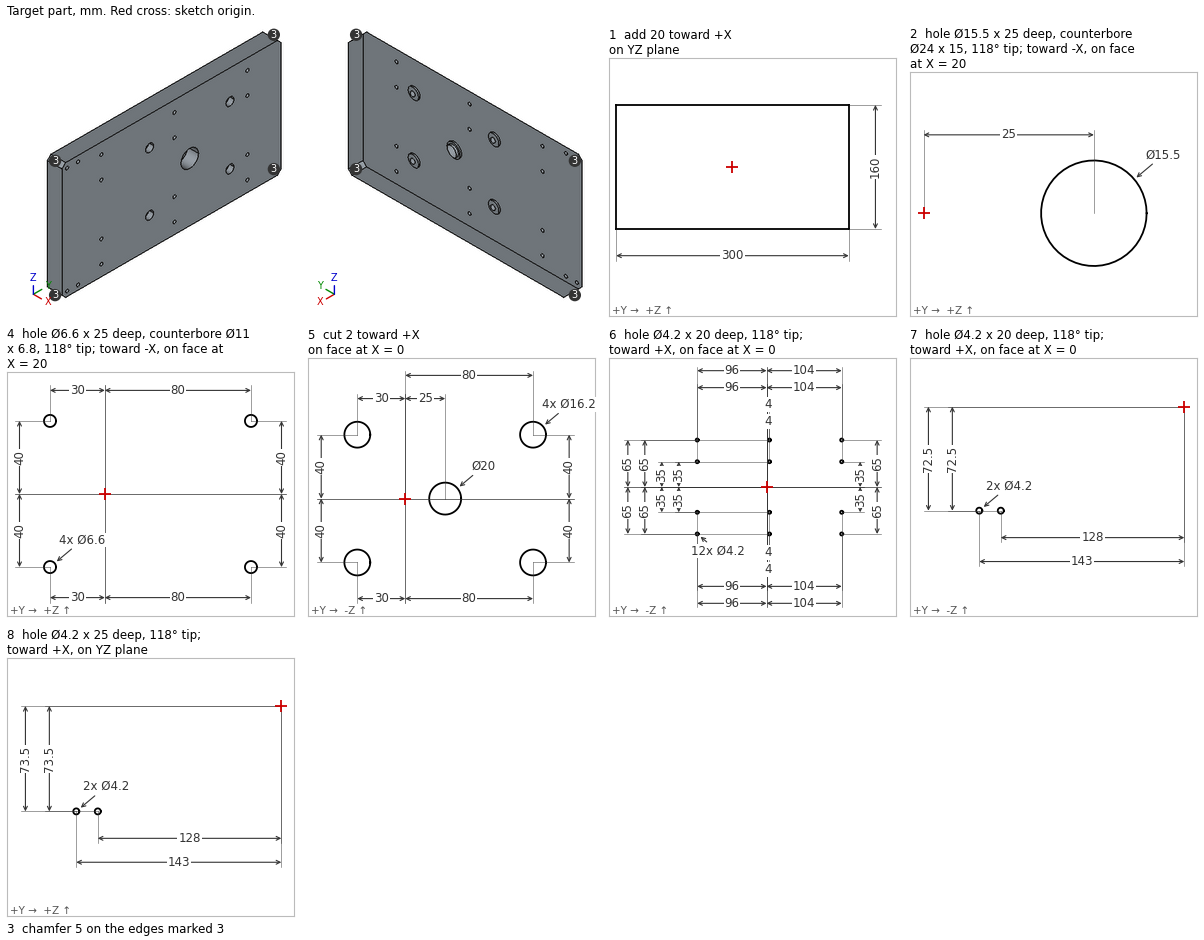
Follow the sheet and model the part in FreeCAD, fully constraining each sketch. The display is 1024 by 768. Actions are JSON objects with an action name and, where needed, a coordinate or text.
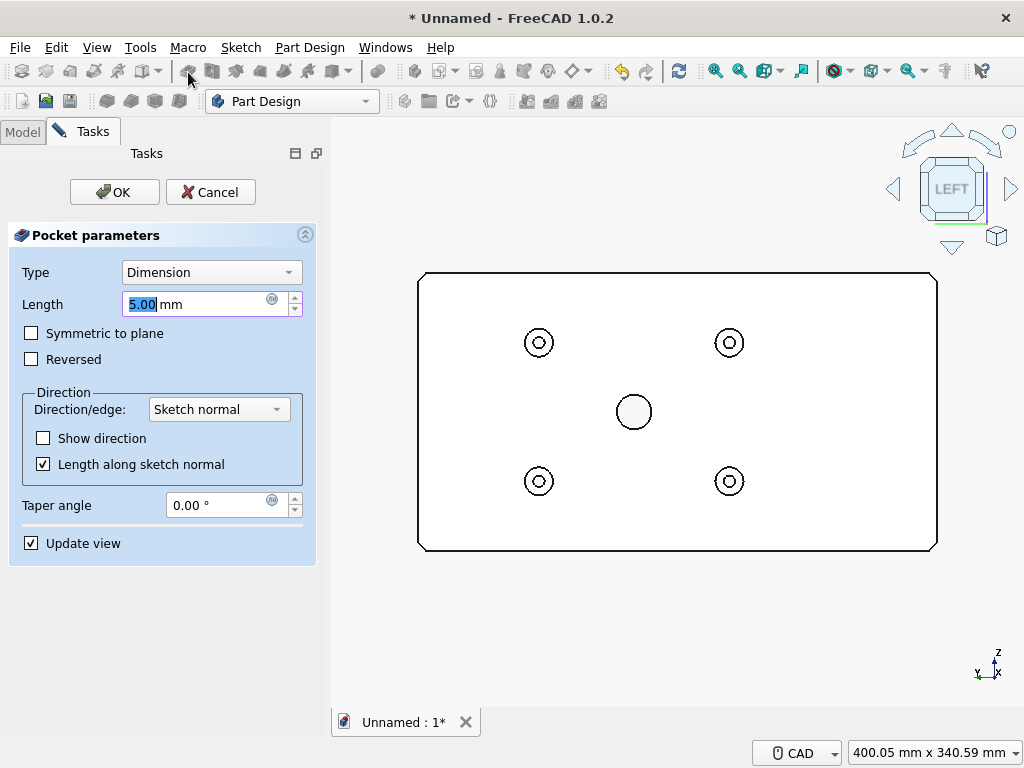
{"action": "type", "text": "2"}
{"action": "key", "text": "Tab"}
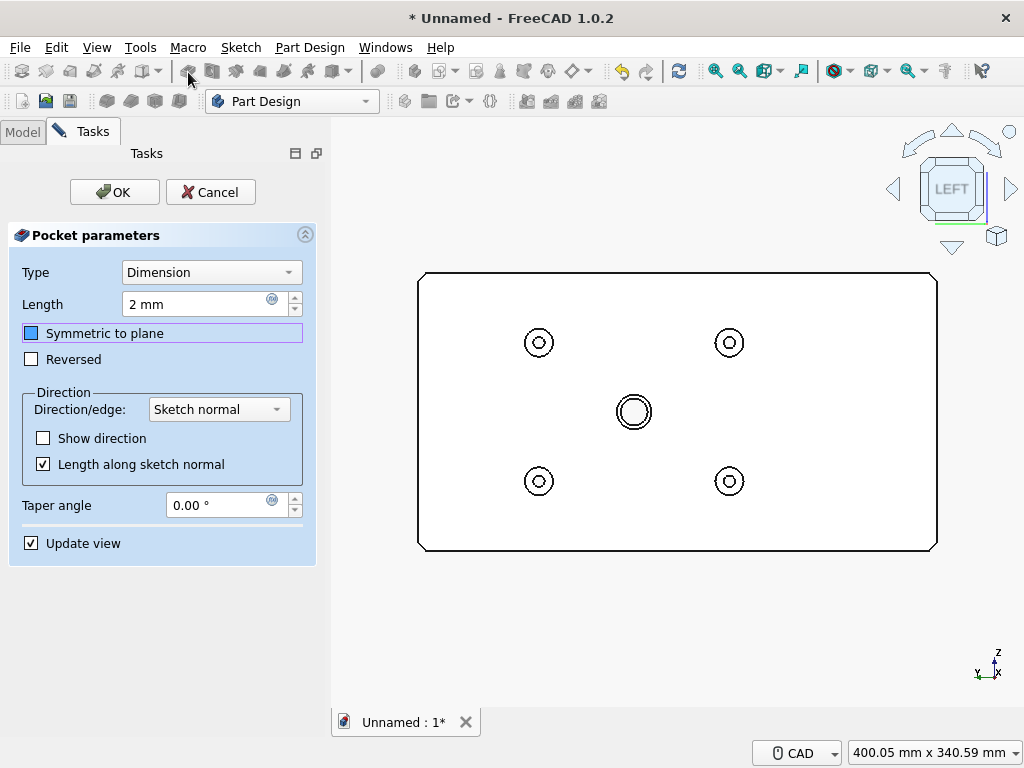
{"action": "left_click", "coordinate": [115, 192]}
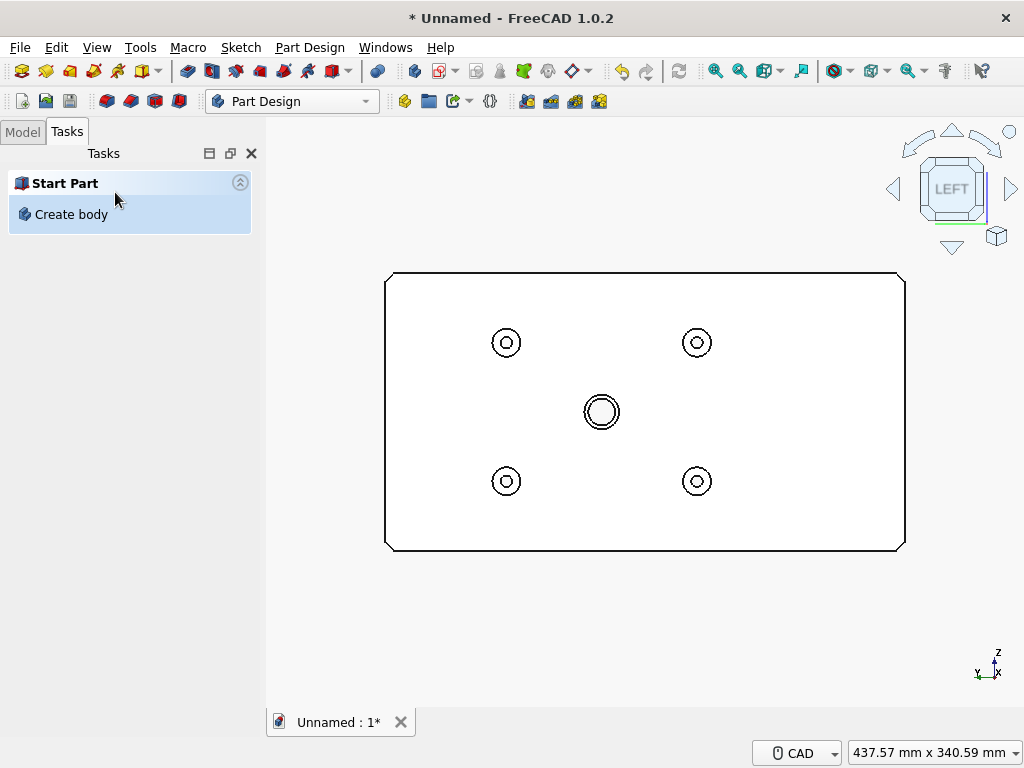
{"action": "left_click", "coordinate": [793, 411]}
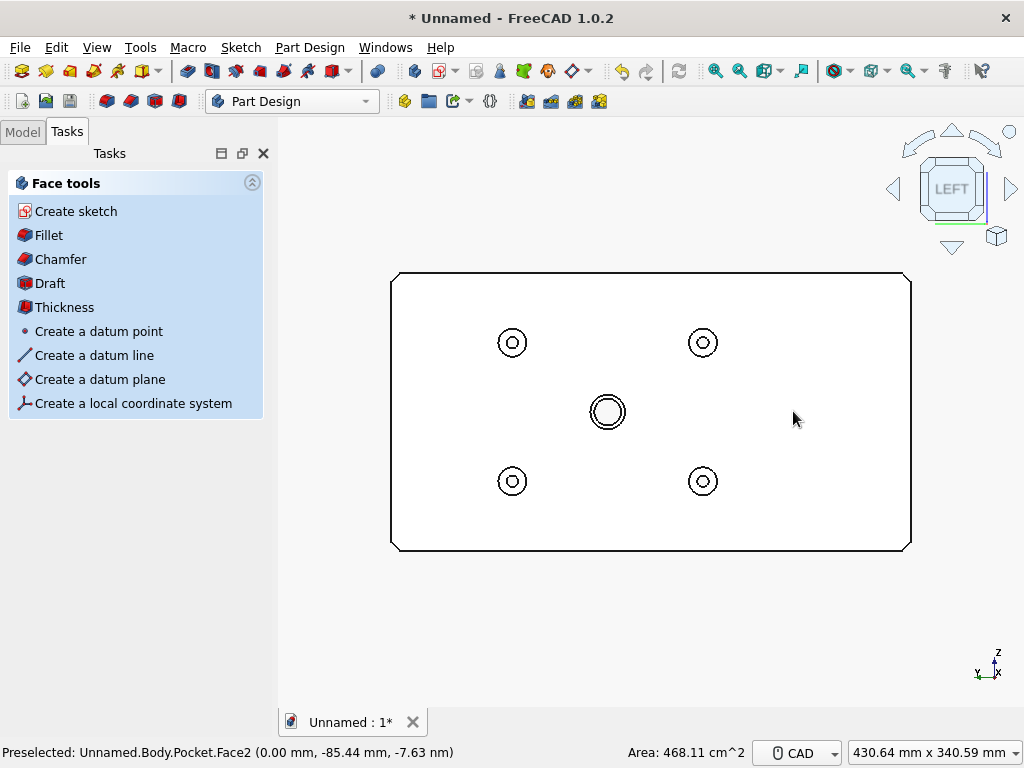
{"action": "left_click", "coordinate": [440, 72]}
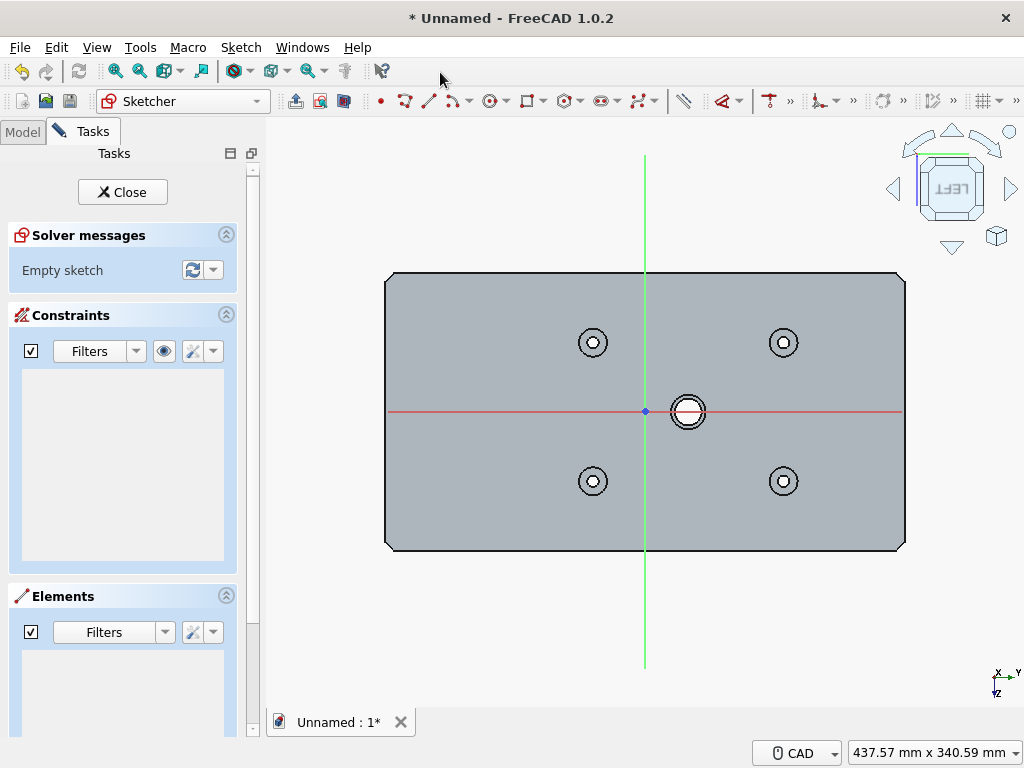
{"action": "left_click", "coordinate": [490, 102]}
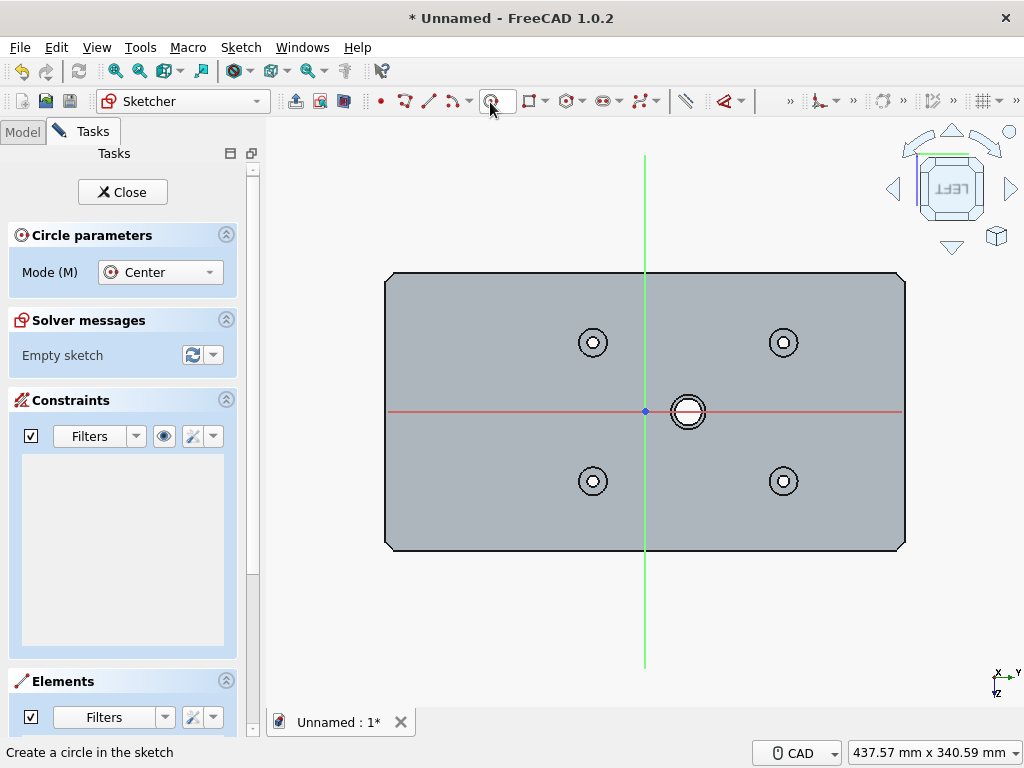
{"action": "scroll", "coordinate": [479, 525], "scroll_direction": "up", "scroll_amount": 10}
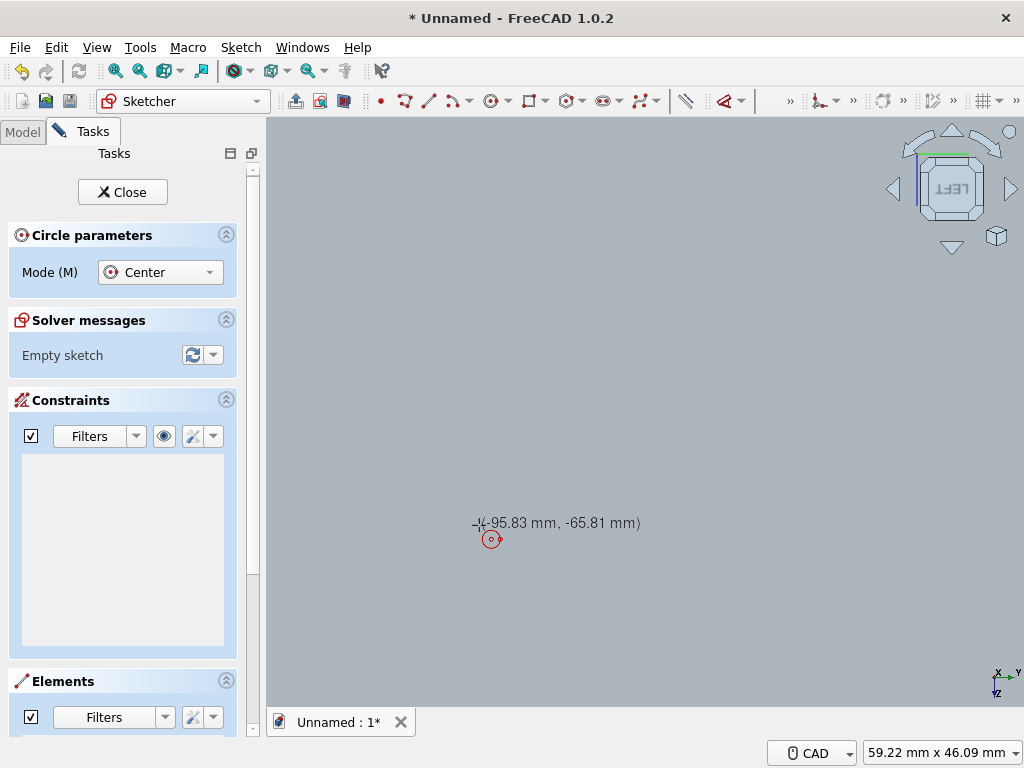
{"action": "scroll", "coordinate": [343, 556], "scroll_direction": "down", "scroll_amount": 9}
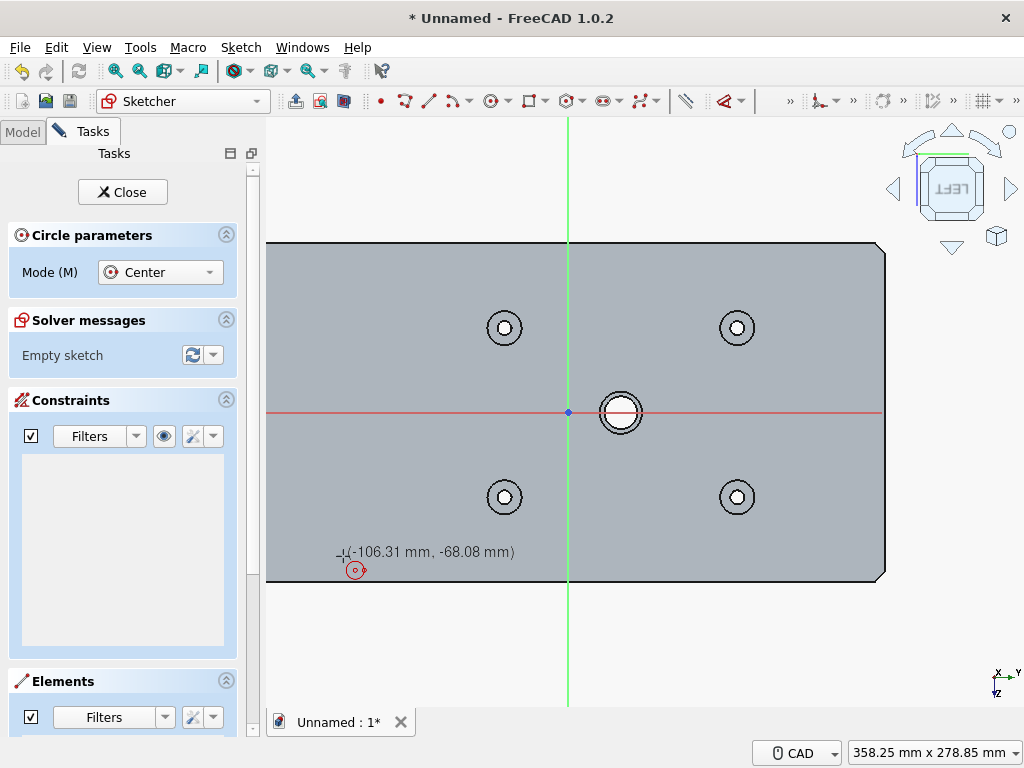
{"action": "left_click", "coordinate": [365, 550]}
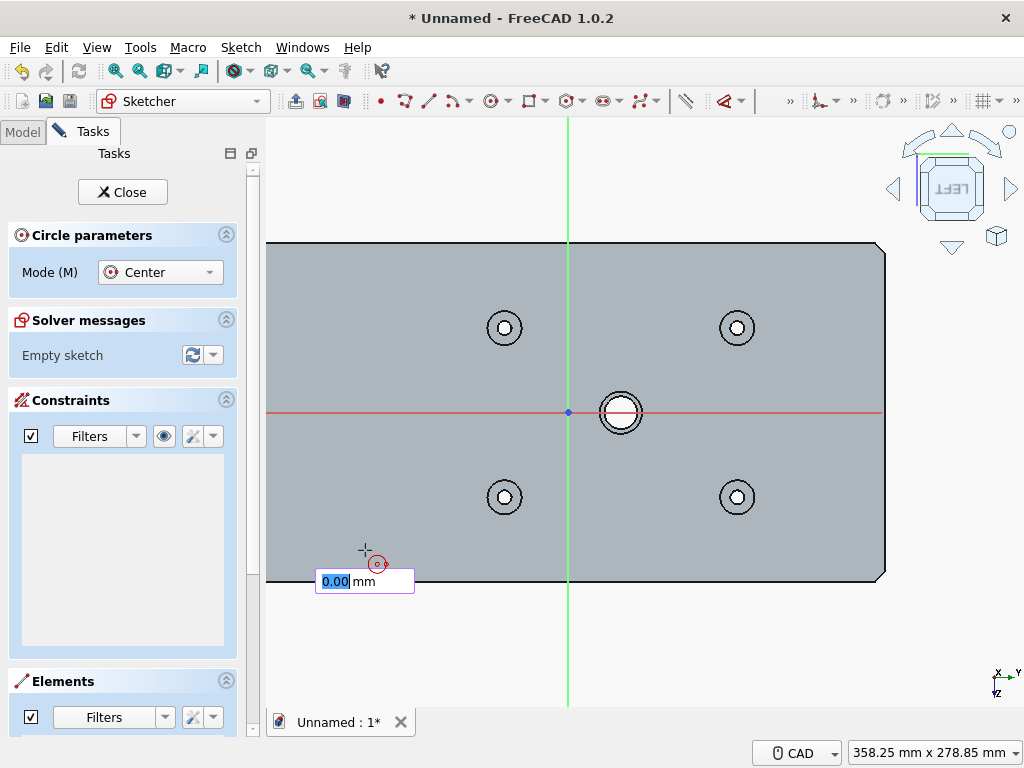
{"action": "scroll", "coordinate": [368, 547], "scroll_direction": "up", "scroll_amount": 7}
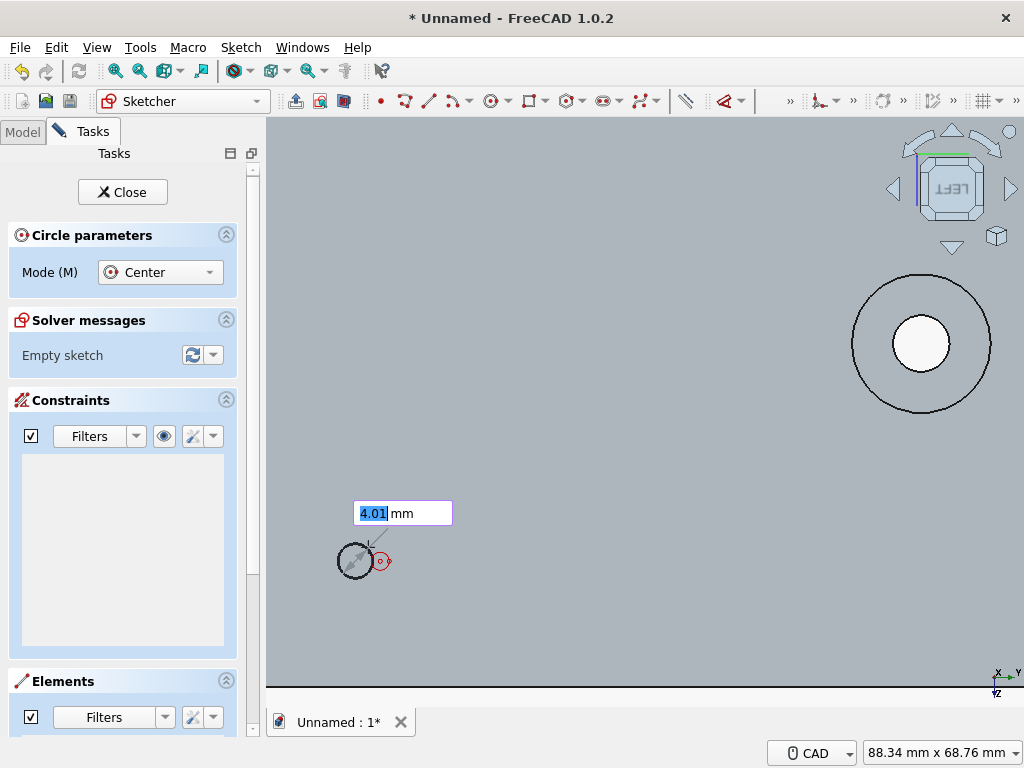
{"action": "left_click", "coordinate": [368, 545]}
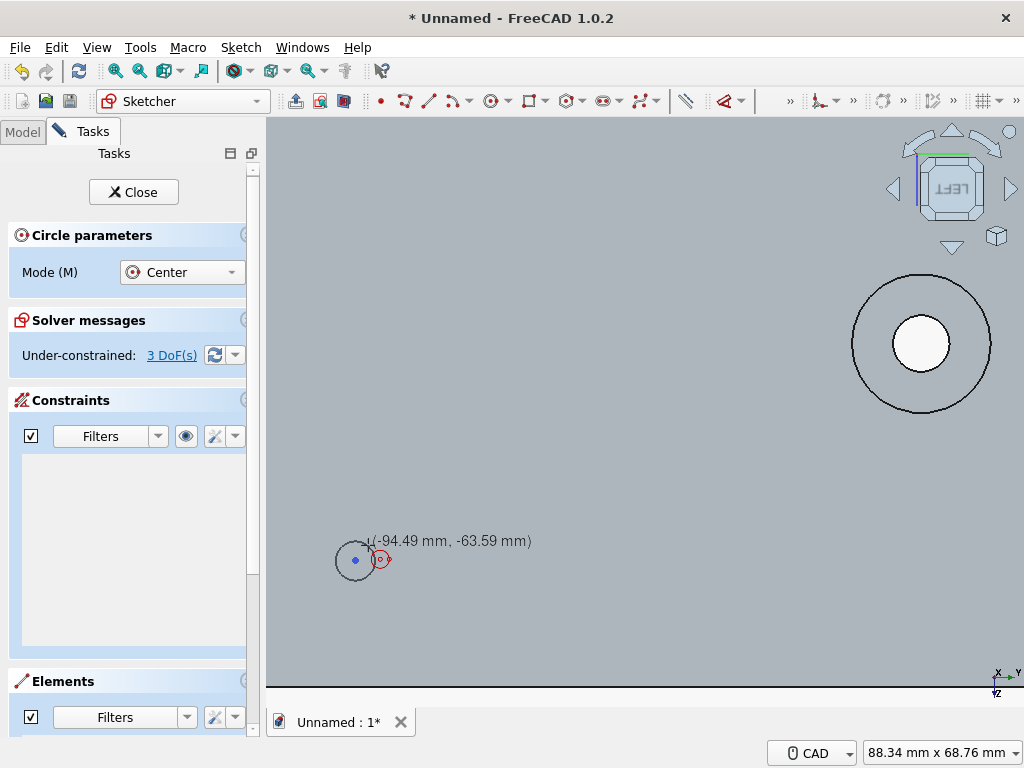
{"action": "scroll", "coordinate": [355, 301], "scroll_direction": "up", "scroll_amount": 2}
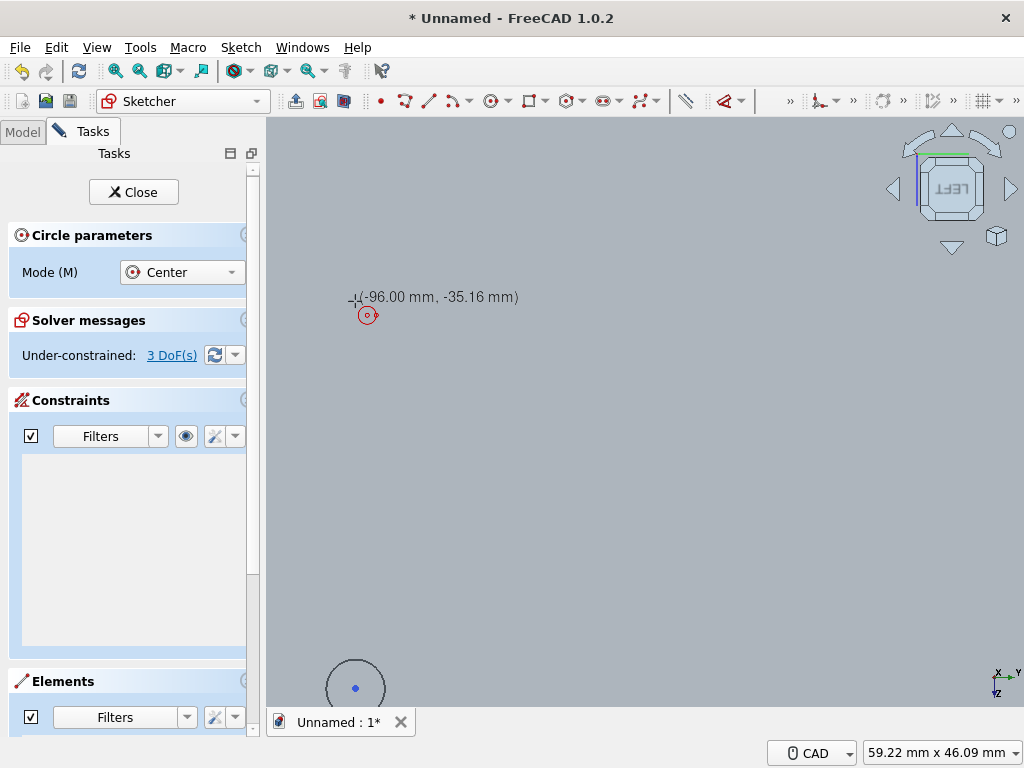
{"action": "scroll", "coordinate": [367, 523], "scroll_direction": "down", "scroll_amount": 9}